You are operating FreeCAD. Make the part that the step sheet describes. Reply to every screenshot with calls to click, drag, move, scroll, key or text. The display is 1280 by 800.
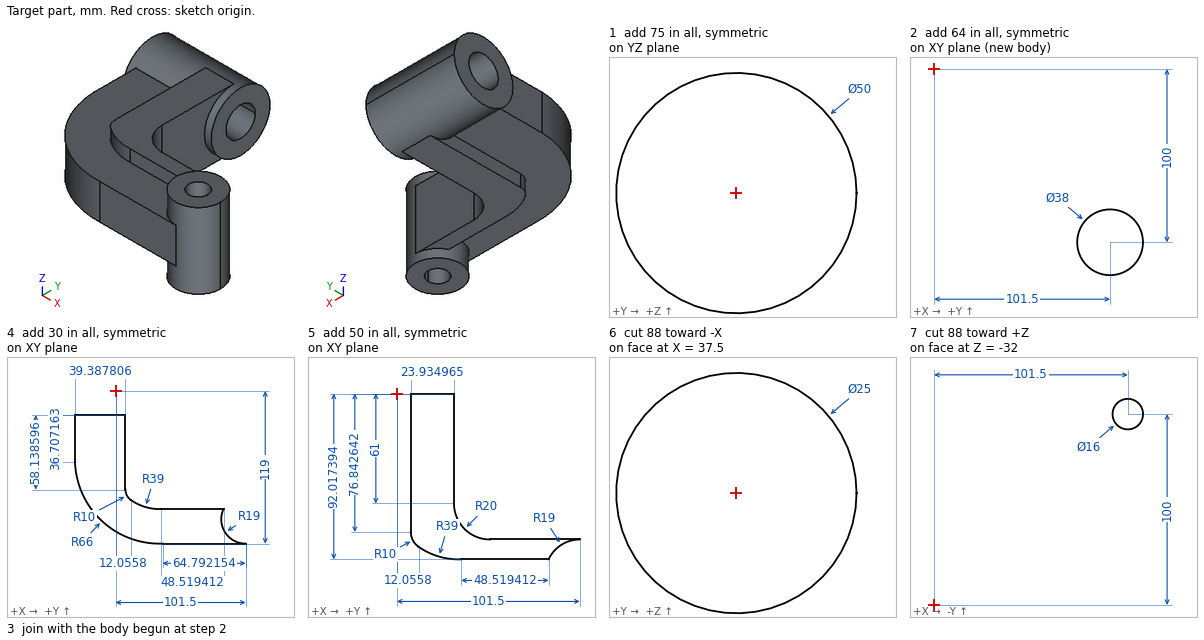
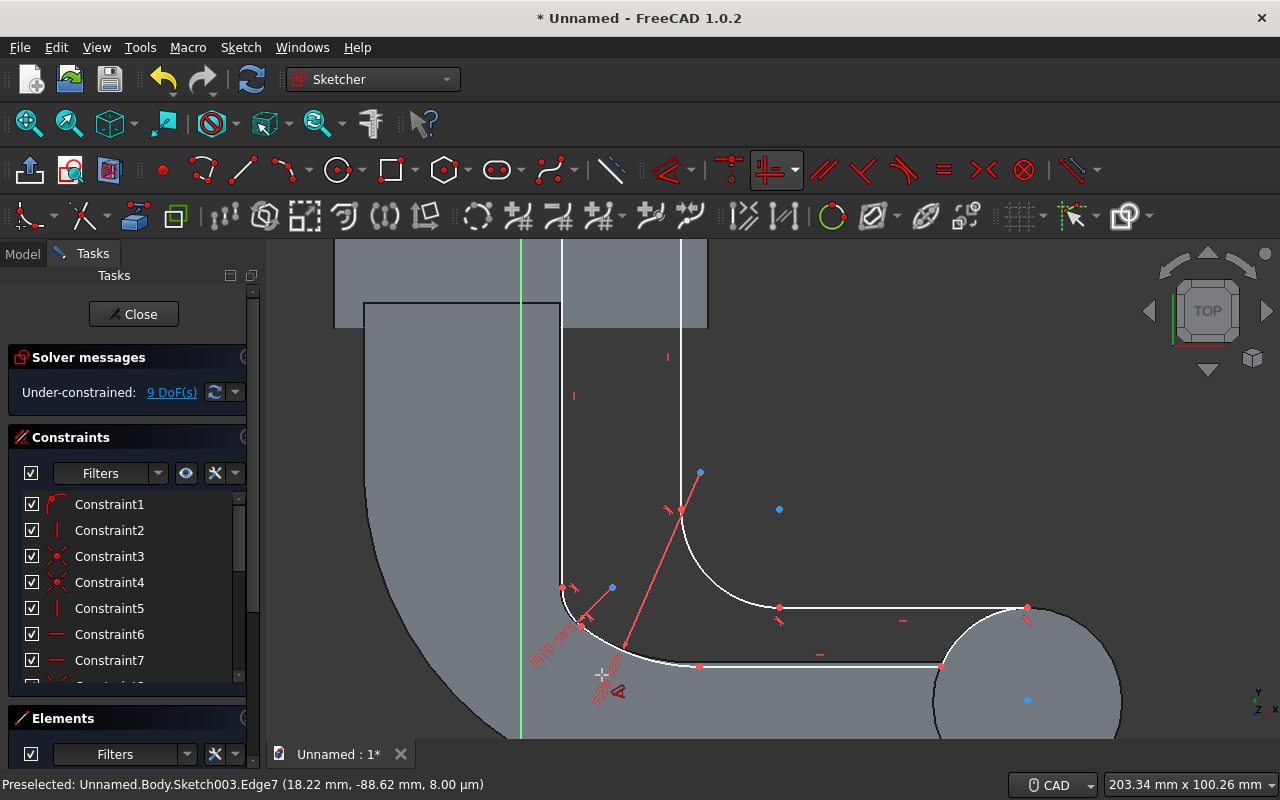
click(959, 639)
click(986, 583)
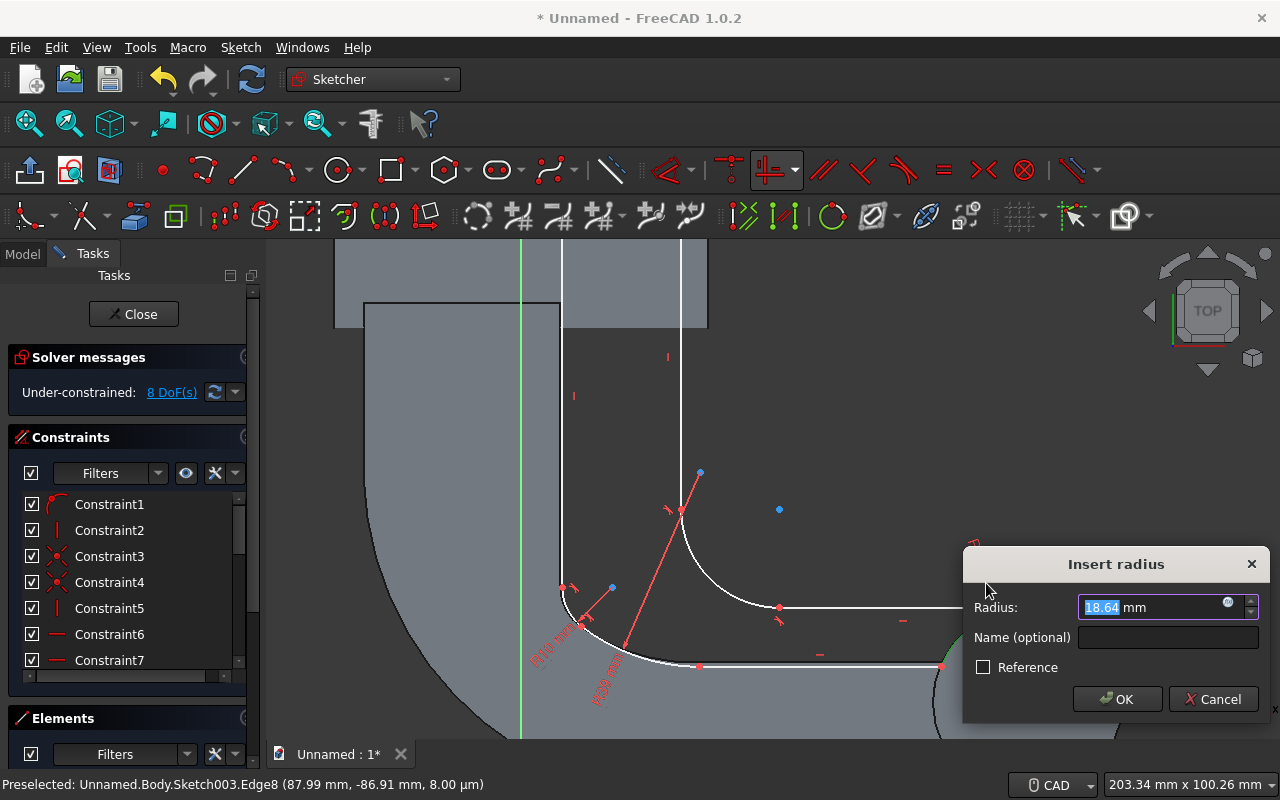
text(19)
key(Return)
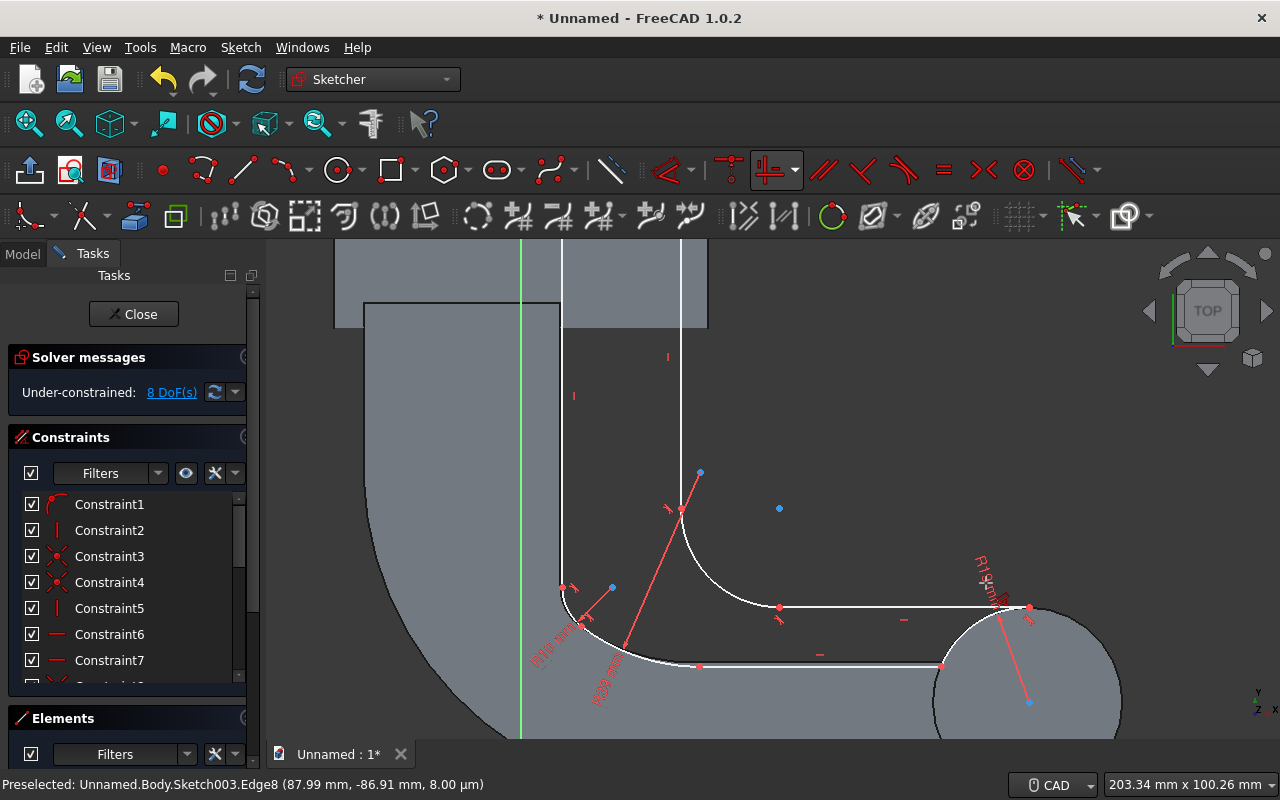
click(692, 553)
click(663, 567)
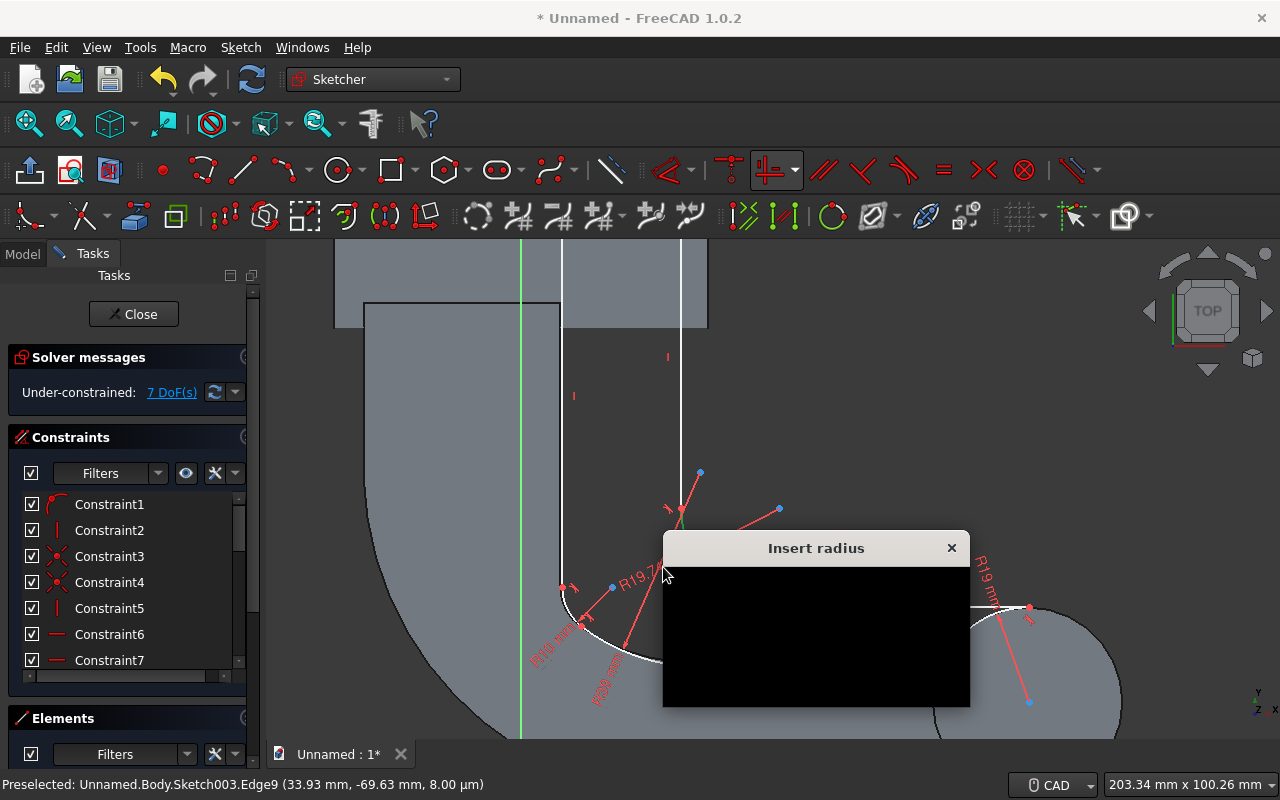
text(20)
key(Return)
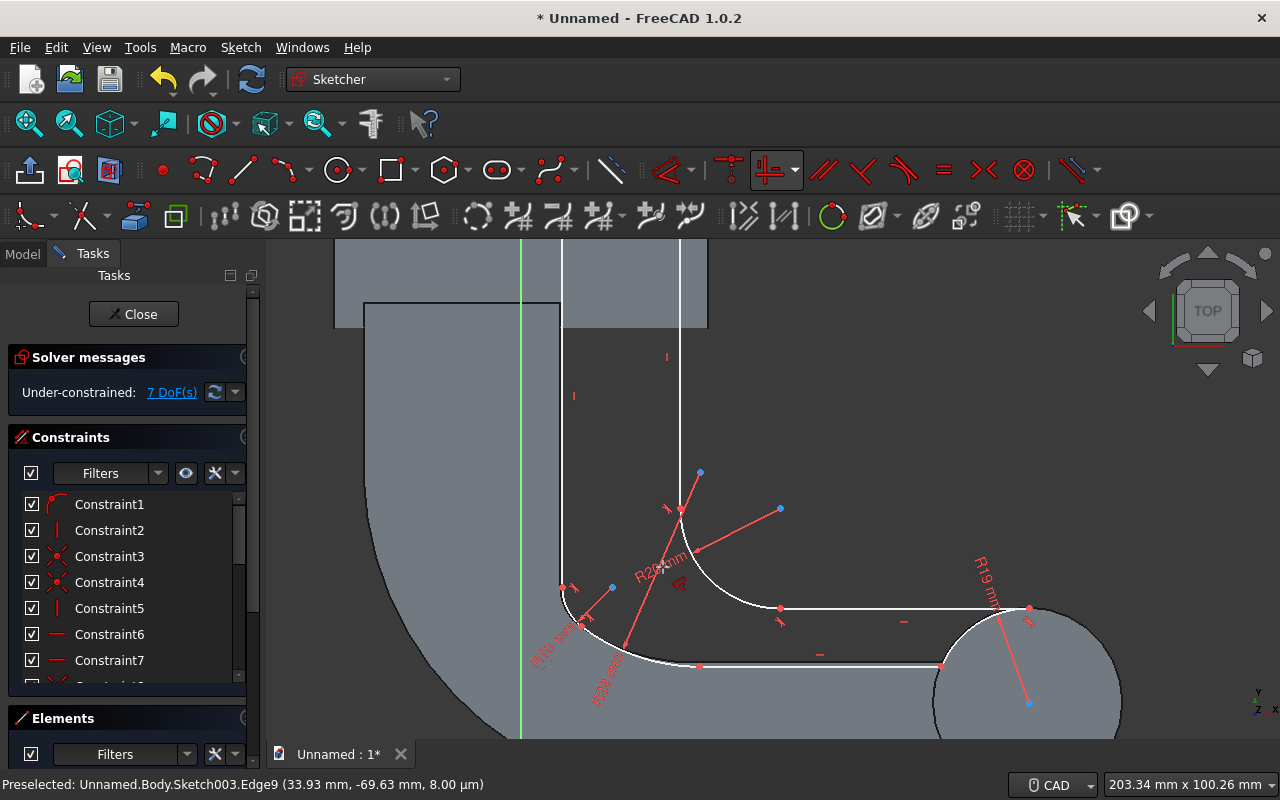
click(680, 417)
click(646, 388)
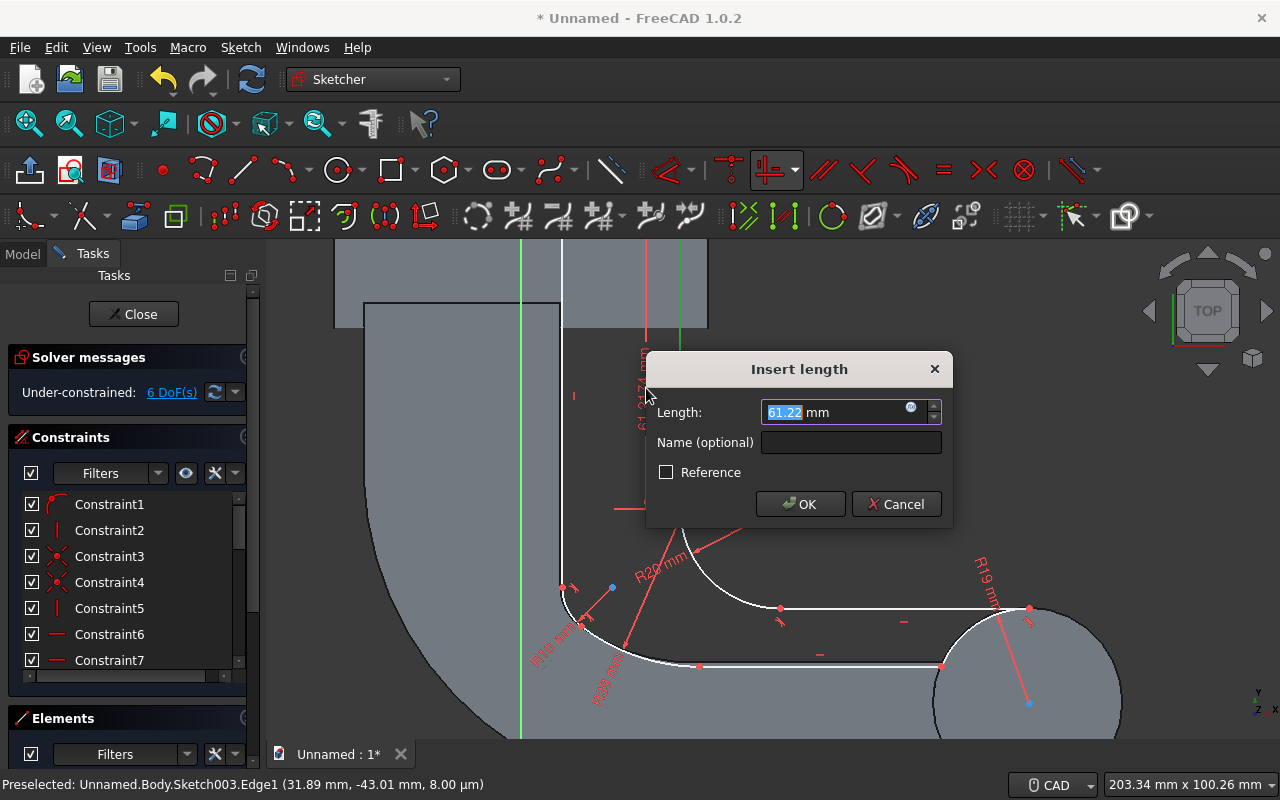
text(61)
key(Return)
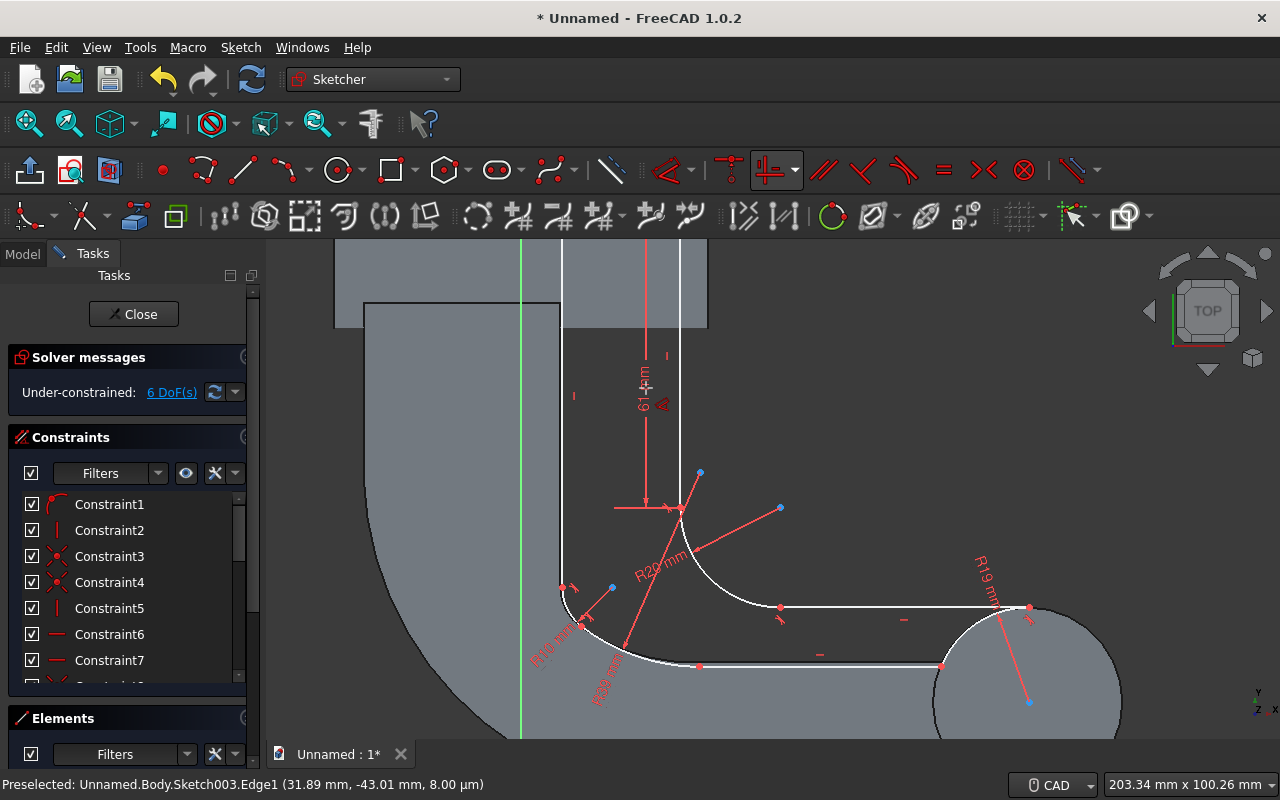
click(1029, 607)
click(775, 641)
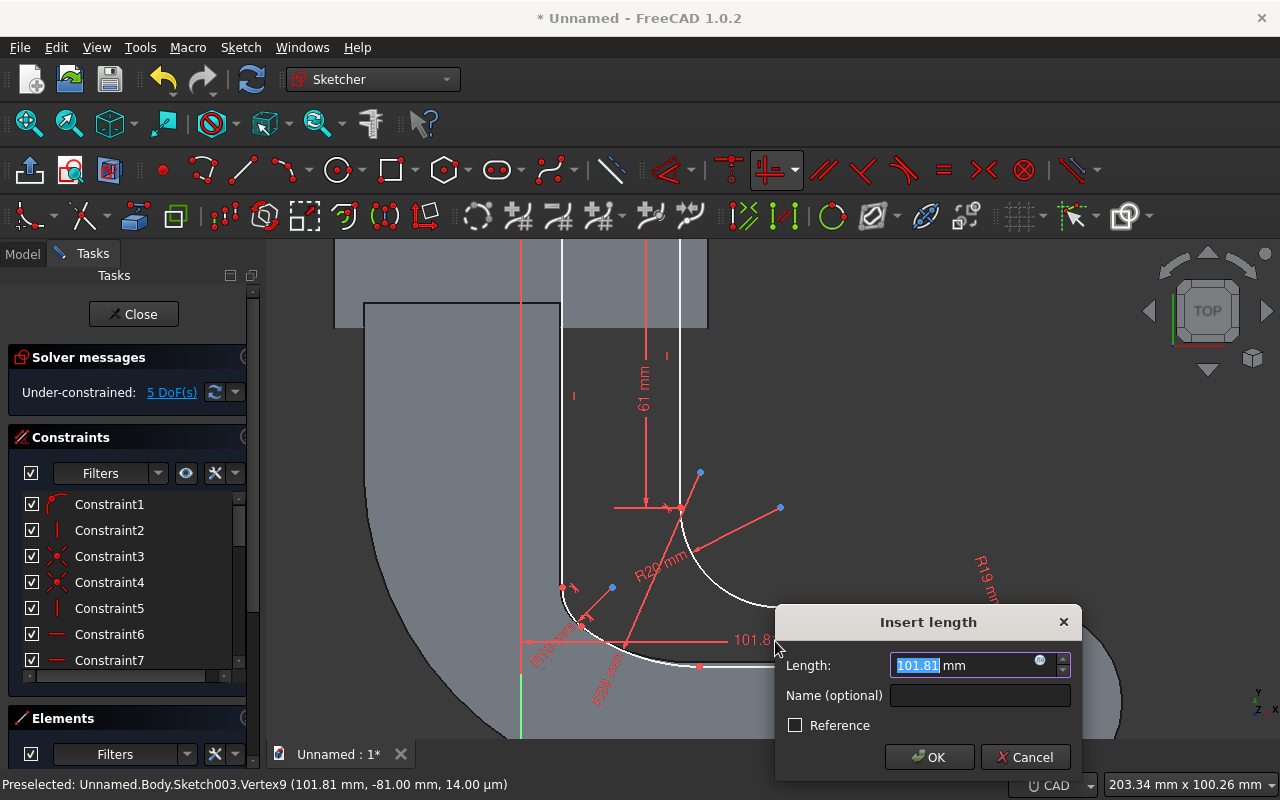
text(101.5)
key(Return)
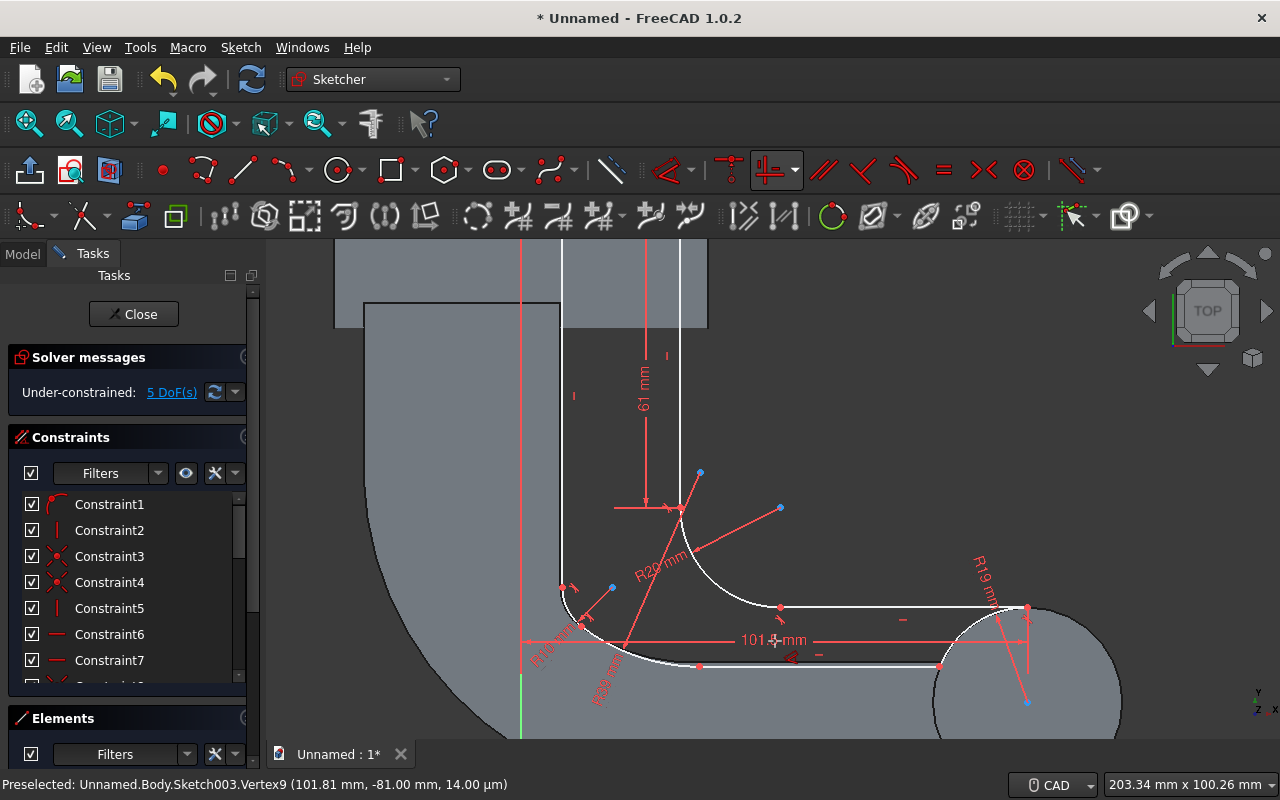
click(582, 627)
click(552, 709)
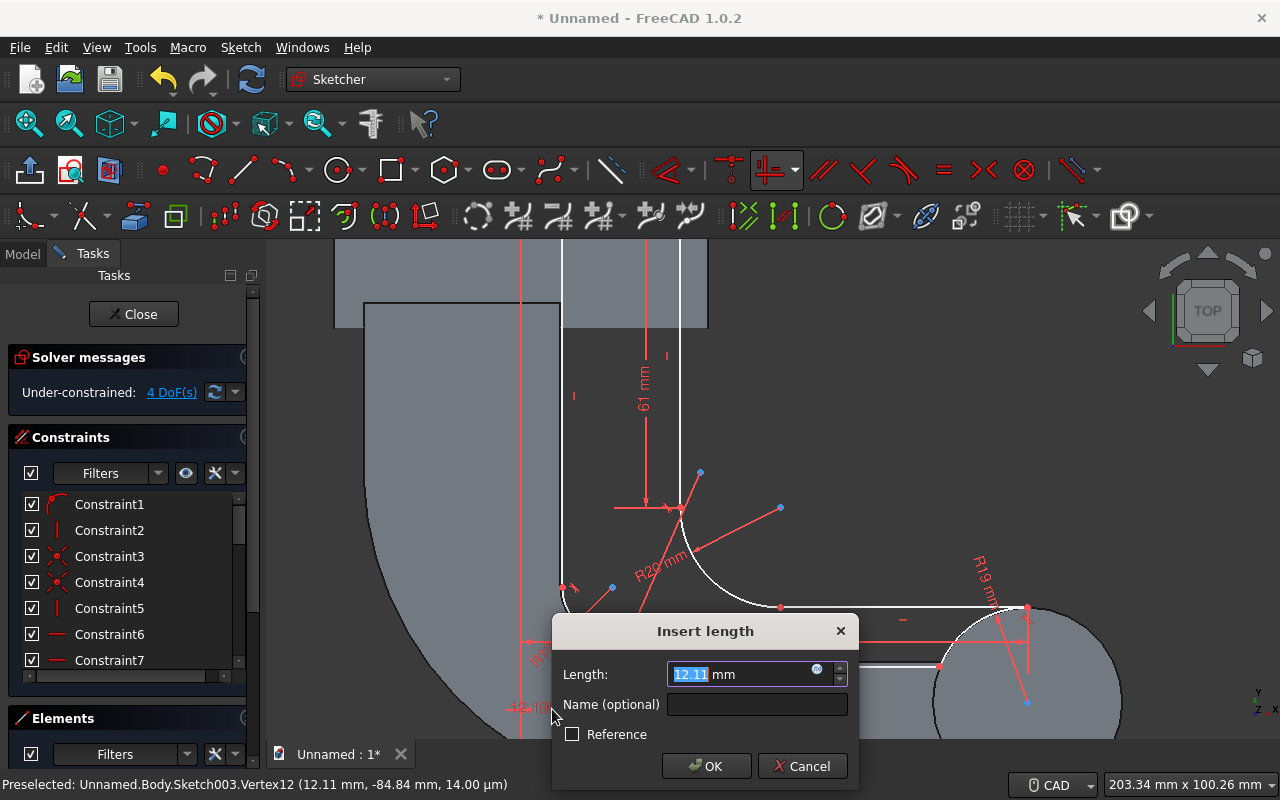
text(12.0558)
key(Return)